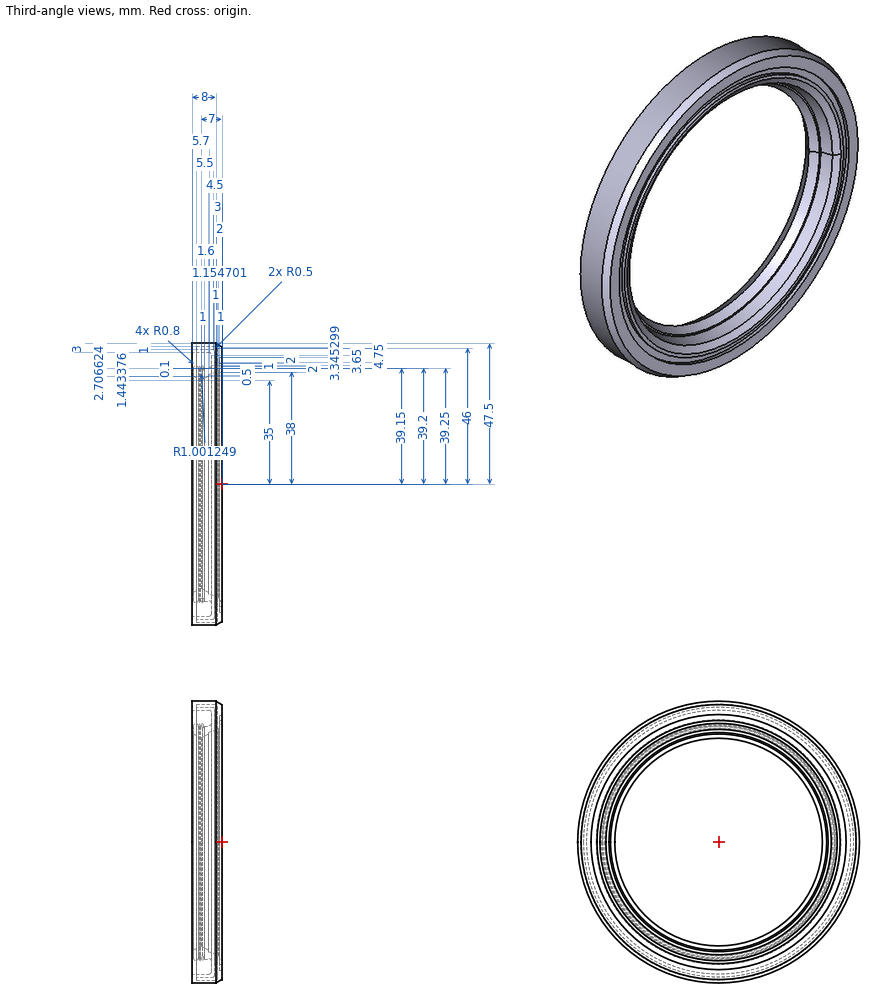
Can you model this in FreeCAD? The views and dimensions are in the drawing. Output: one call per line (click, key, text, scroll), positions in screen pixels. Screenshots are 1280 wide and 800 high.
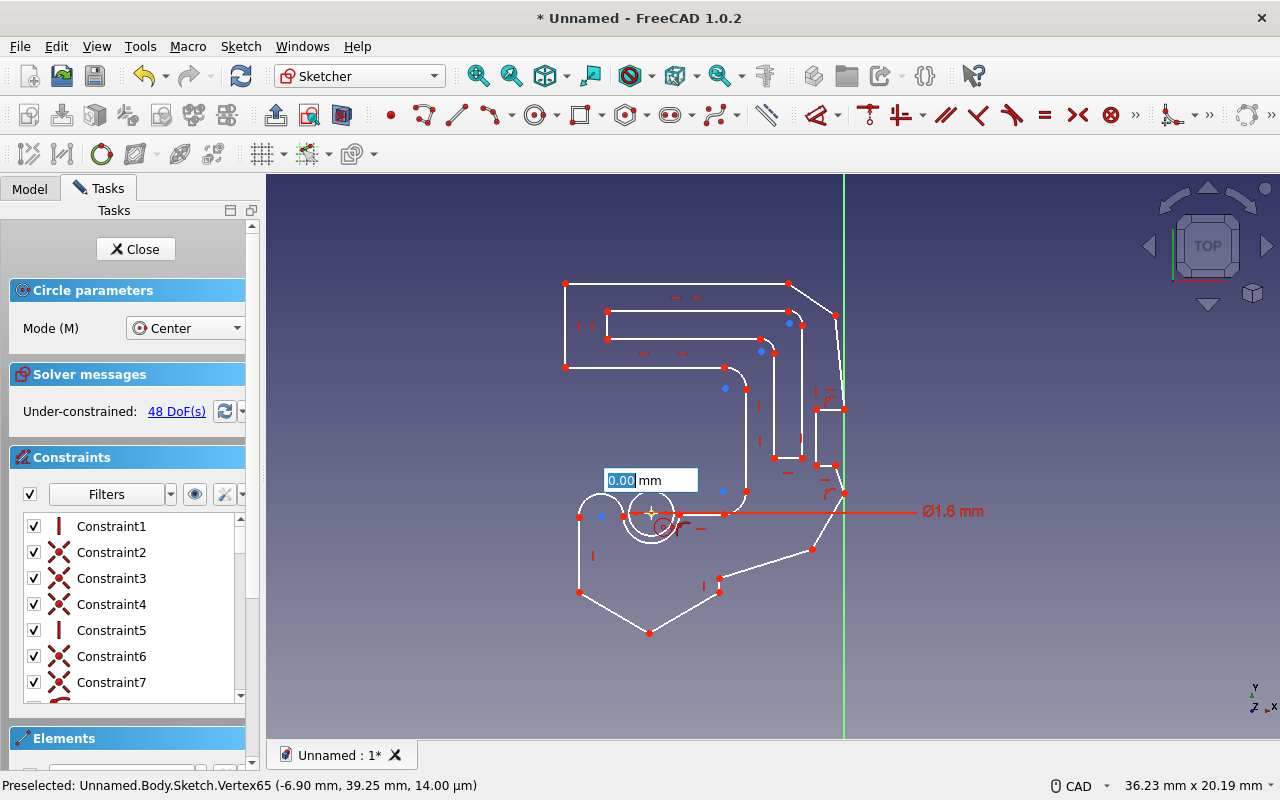
scroll(657, 507, up, 4)
move(657, 507)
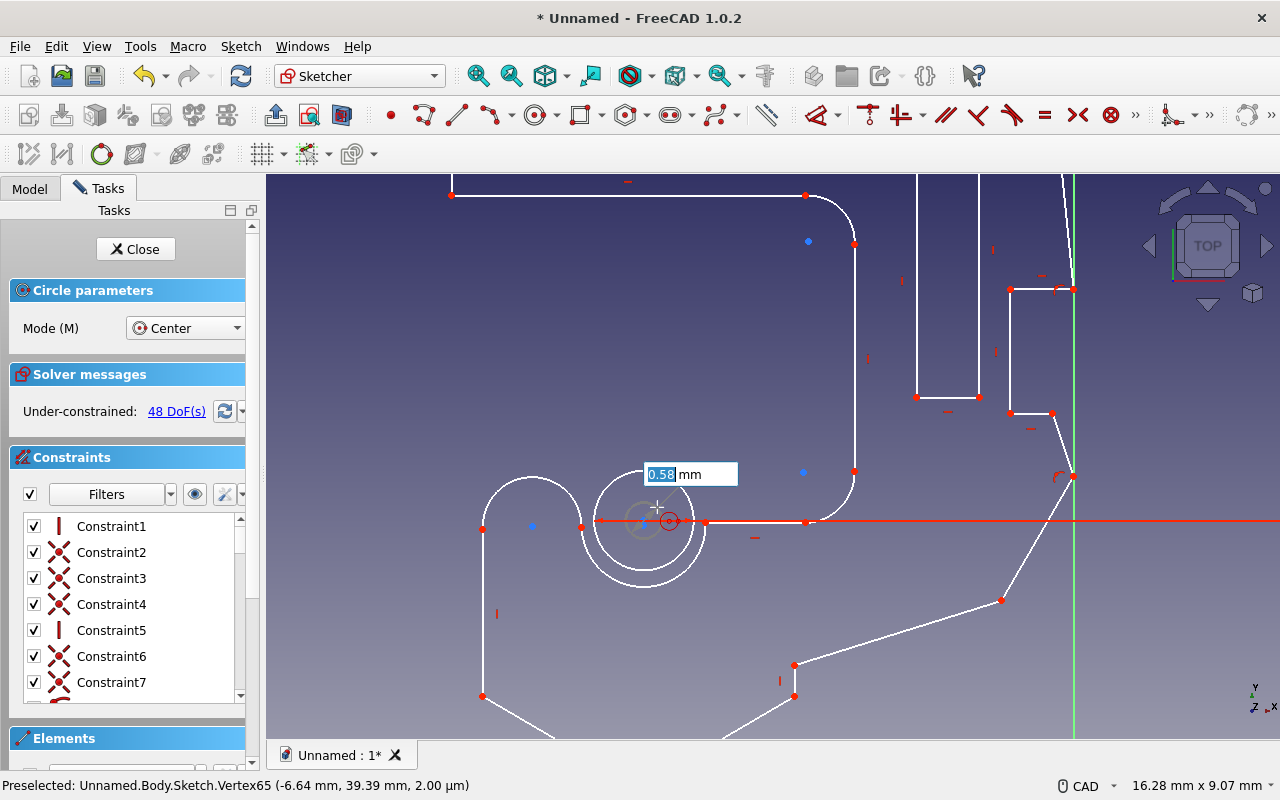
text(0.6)
key(Return)
key(Escape)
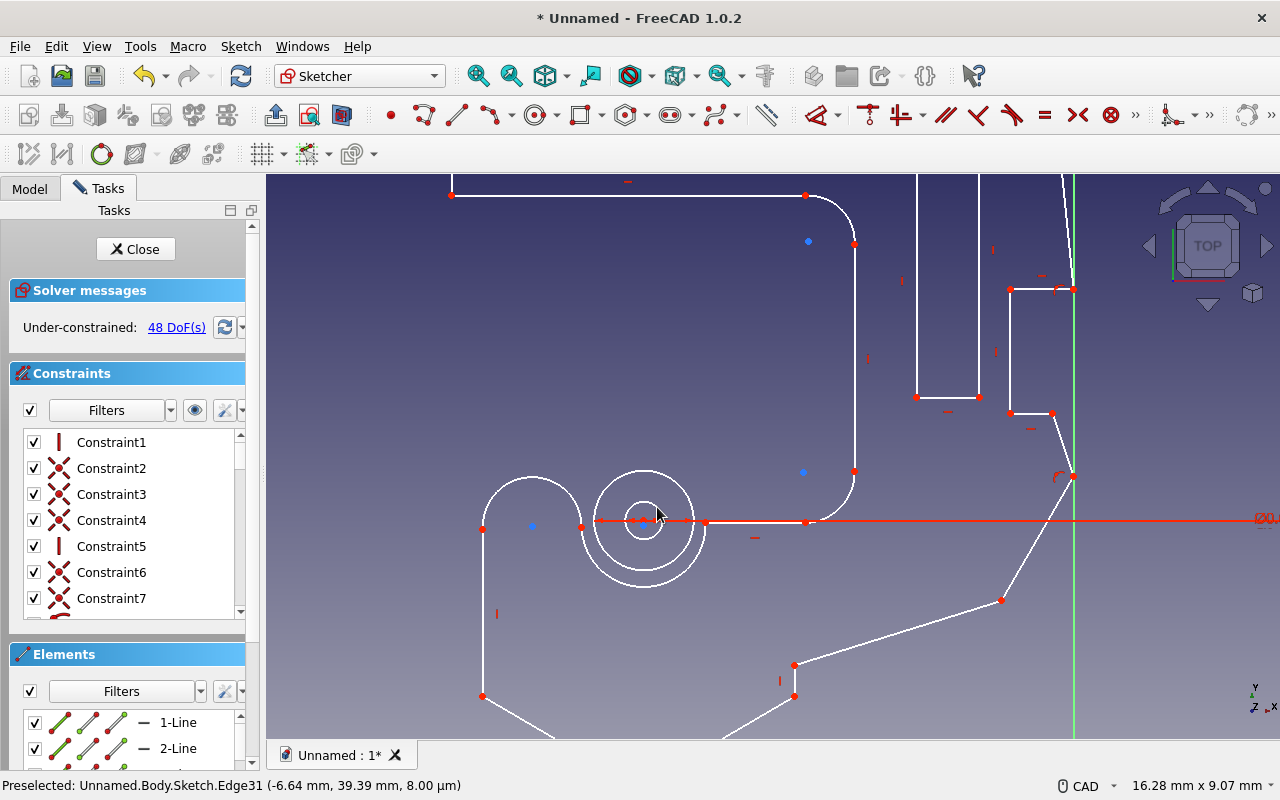
click(483, 580)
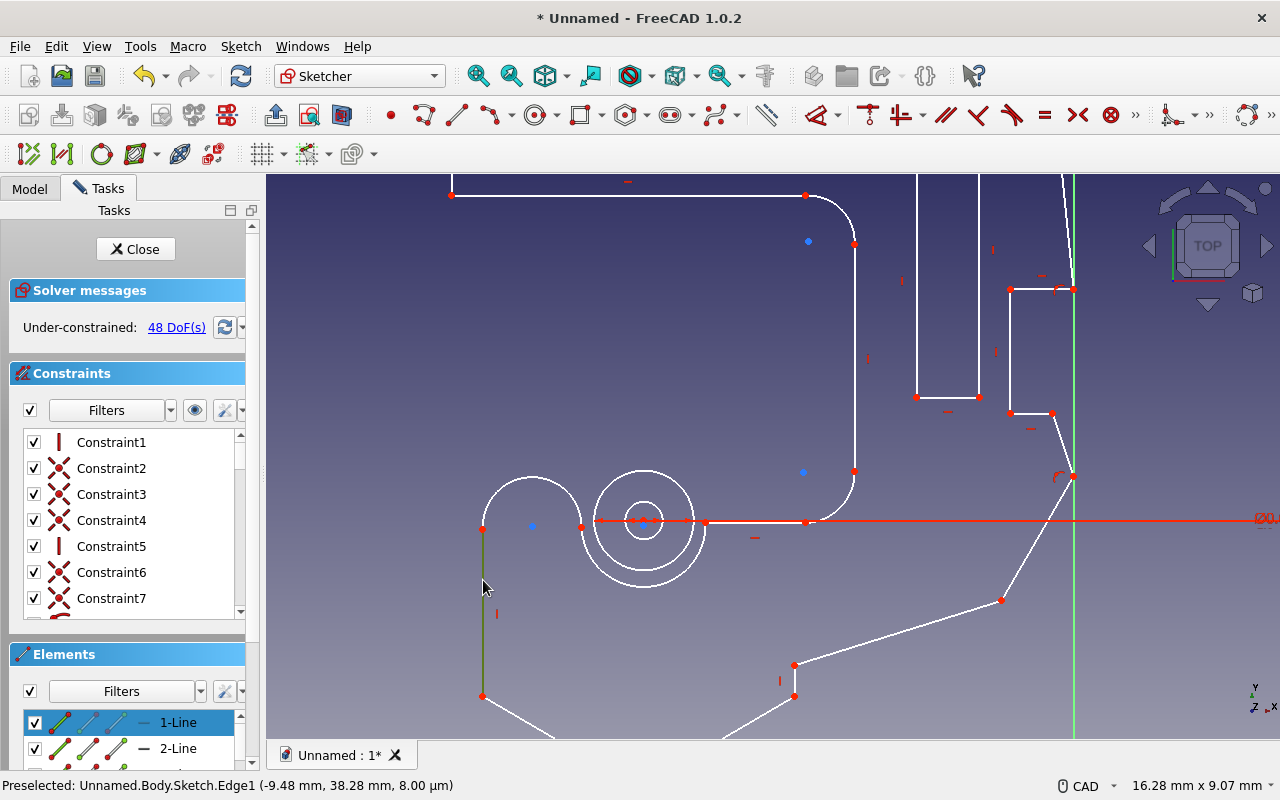
click(561, 486)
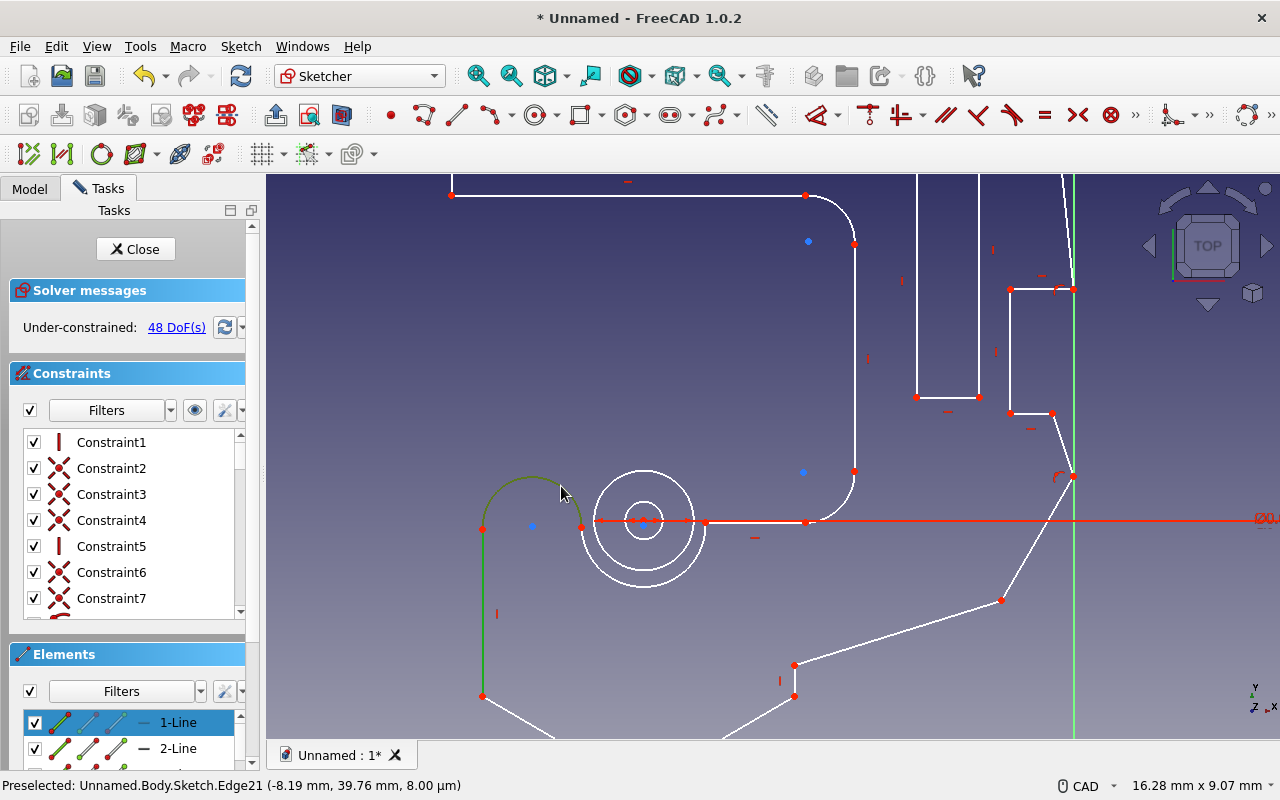
click(1012, 116)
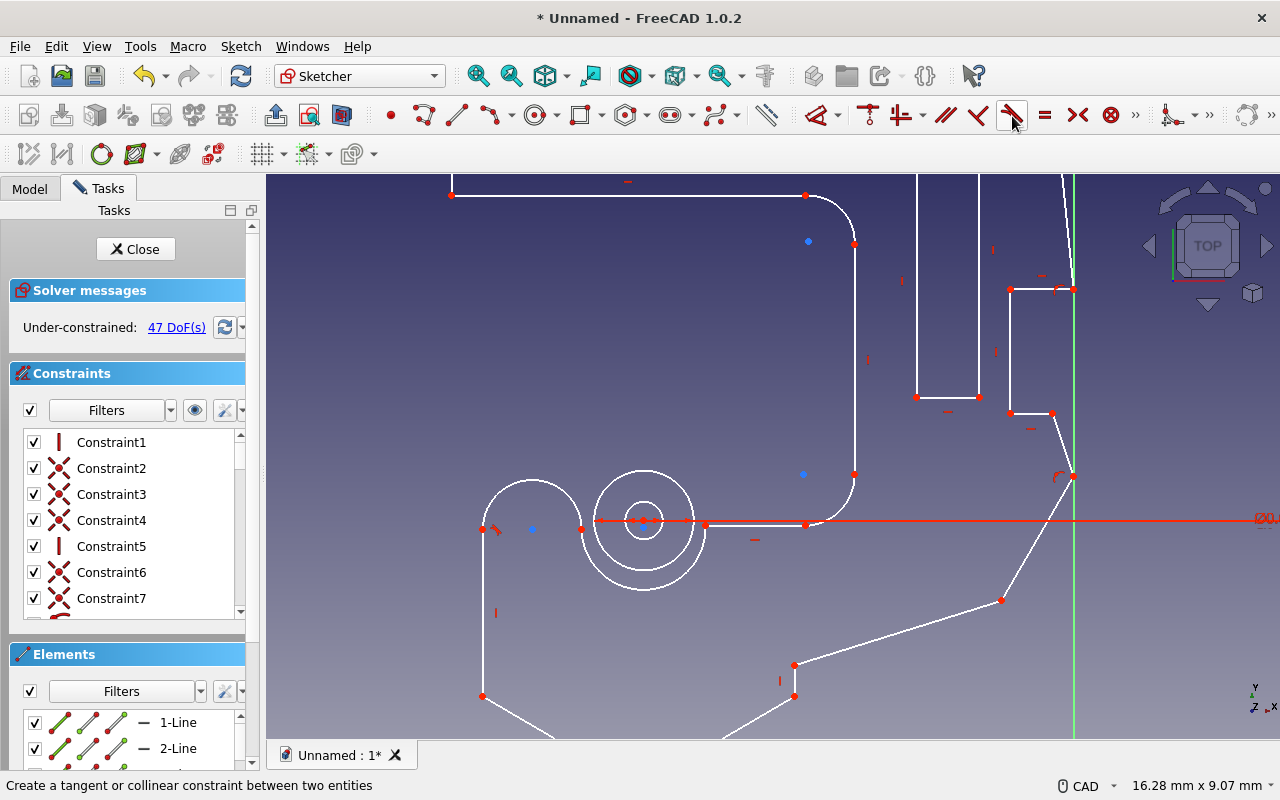
scroll(657, 506, down, 4)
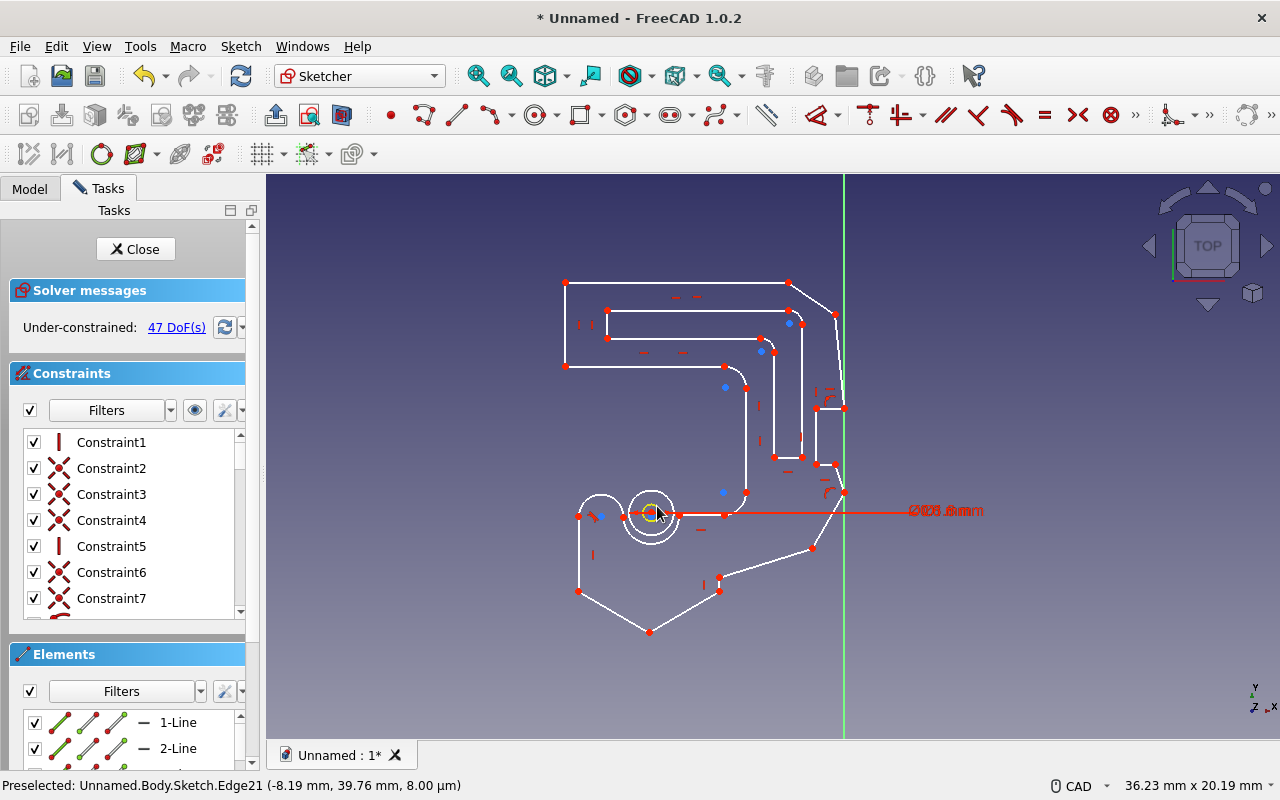
click(613, 367)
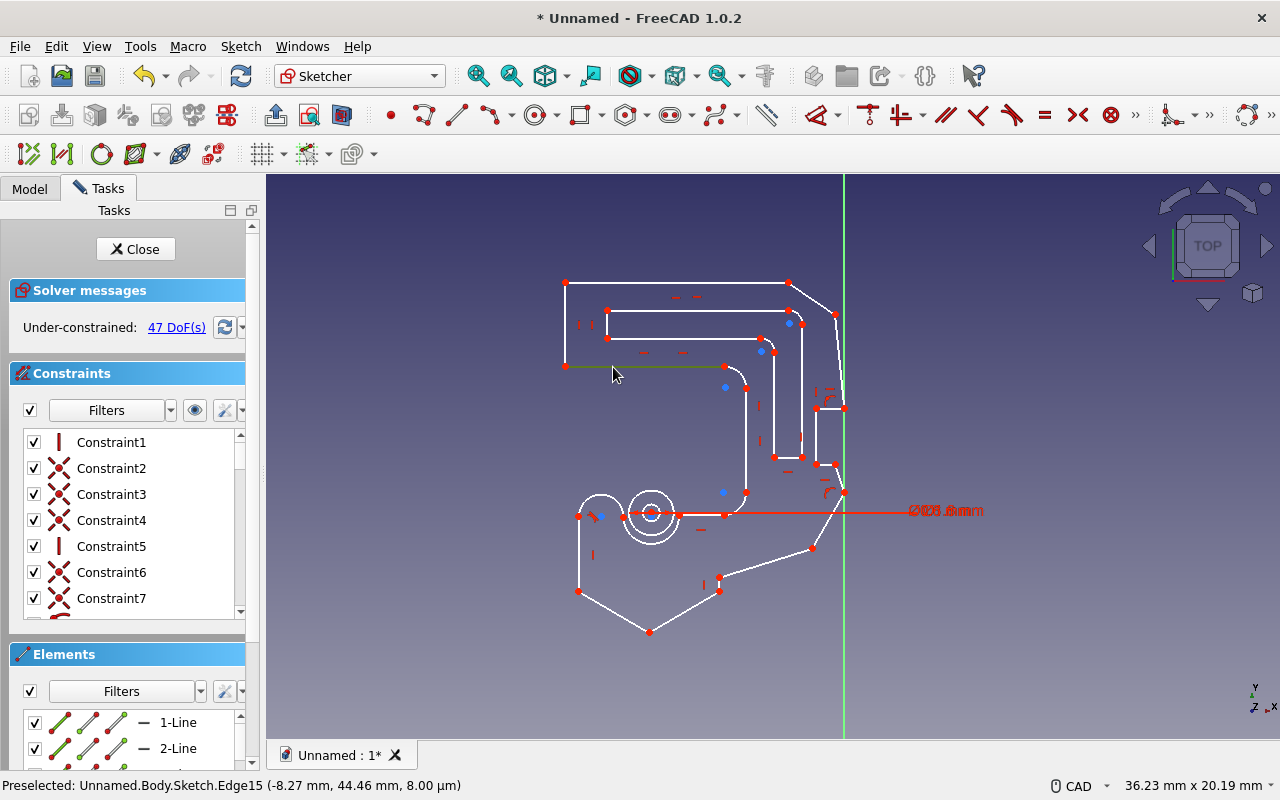
scroll(744, 379, up, 2)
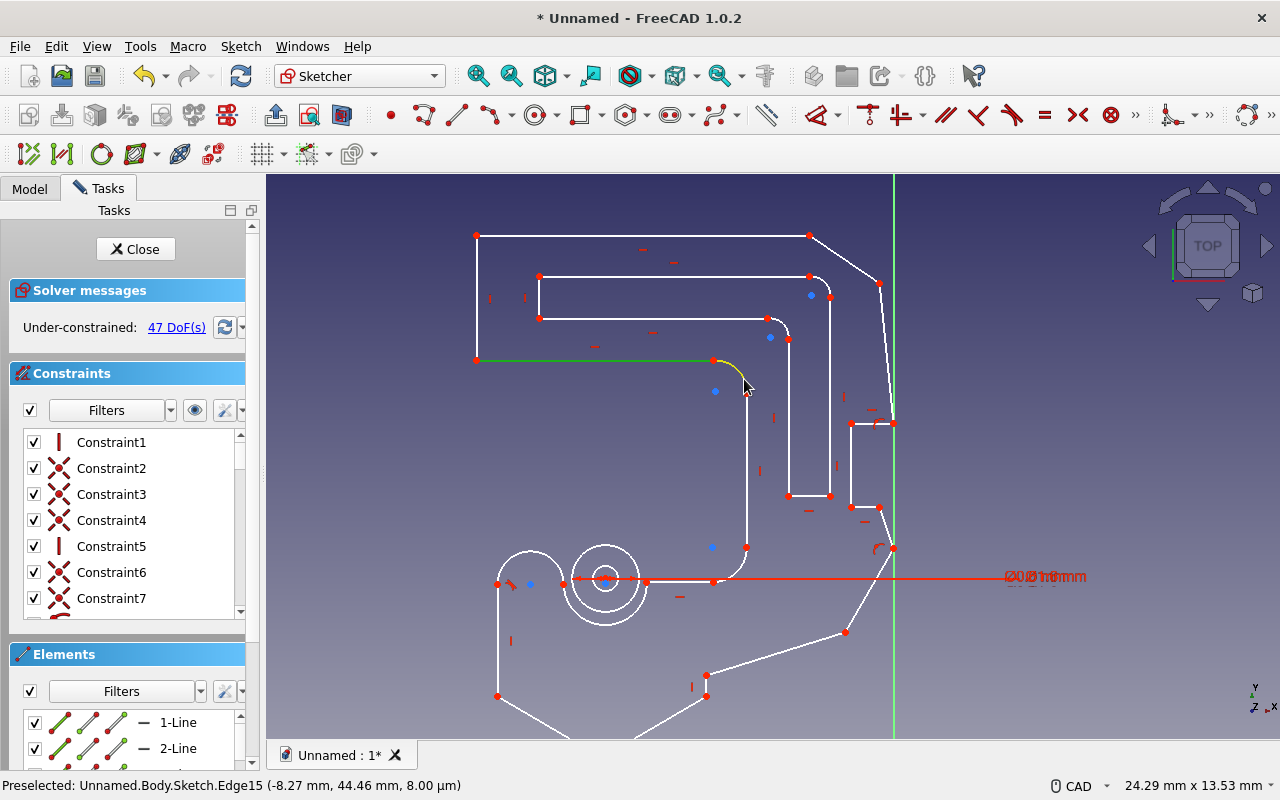
click(744, 378)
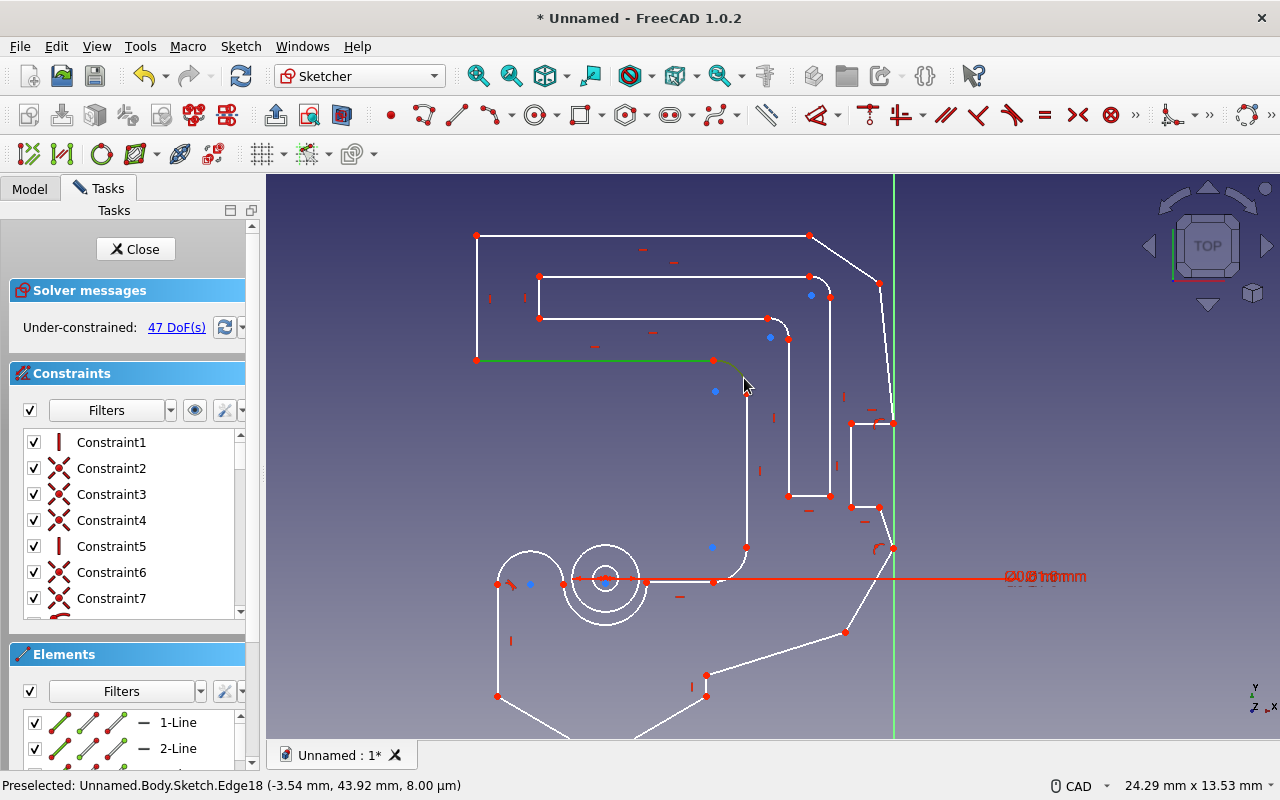
click(1012, 116)